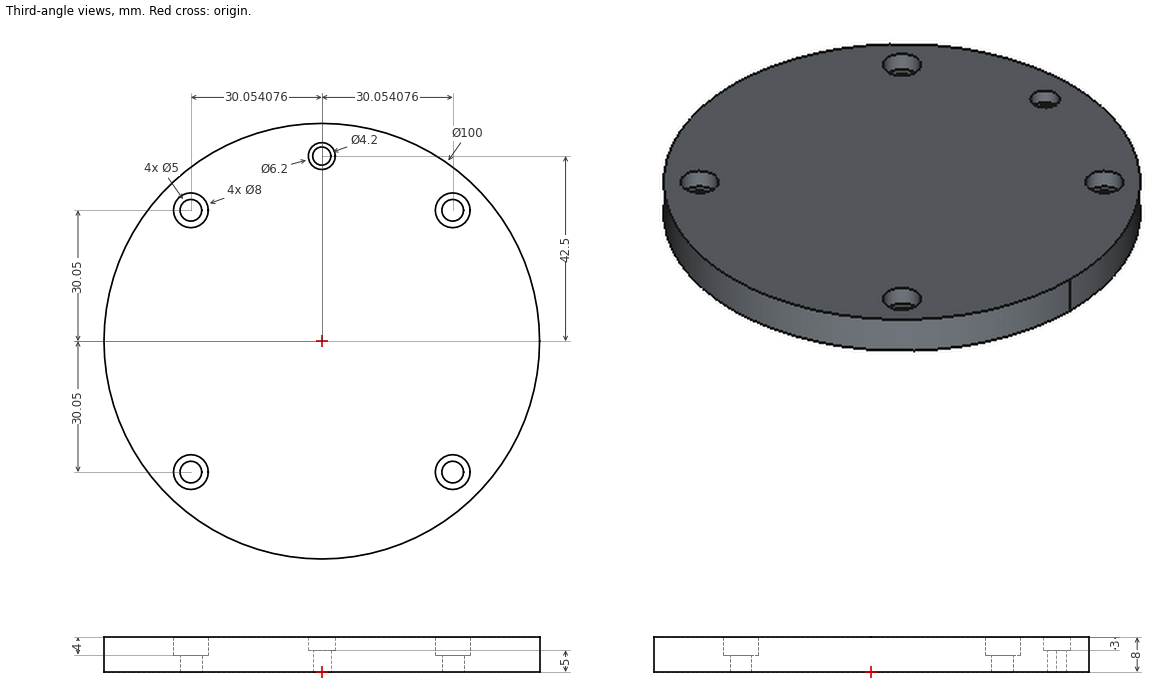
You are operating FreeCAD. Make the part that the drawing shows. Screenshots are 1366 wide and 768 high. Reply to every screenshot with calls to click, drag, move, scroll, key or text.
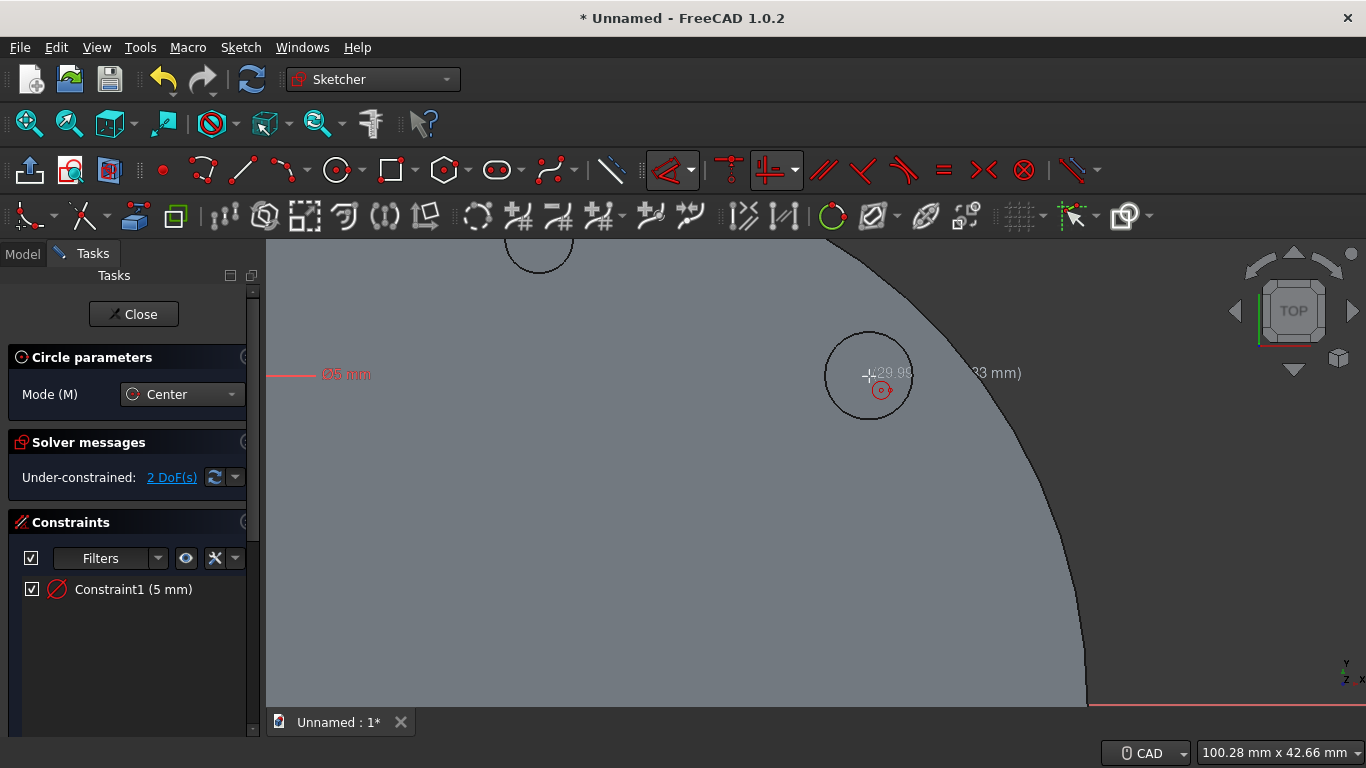
click(869, 376)
move(888, 356)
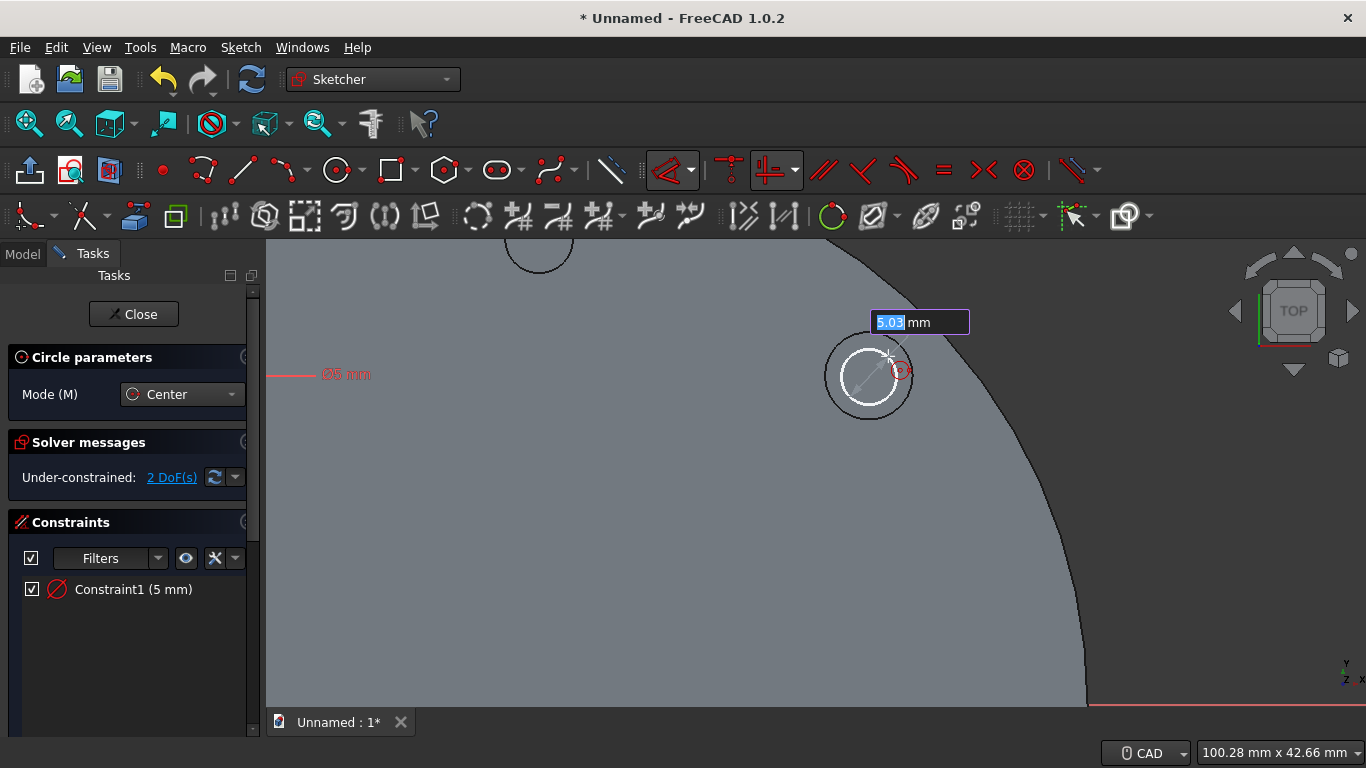
text(5)
key(Return)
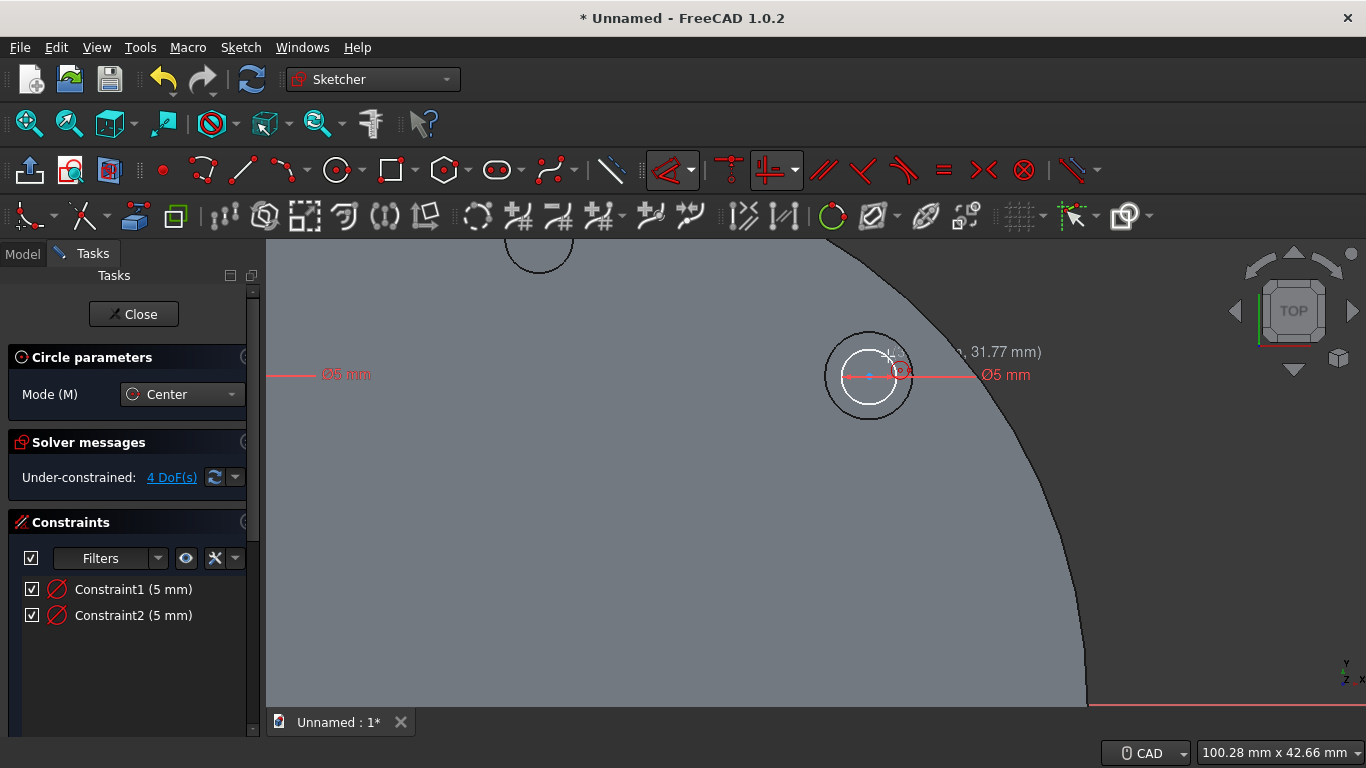
scroll(869, 376, down, 5)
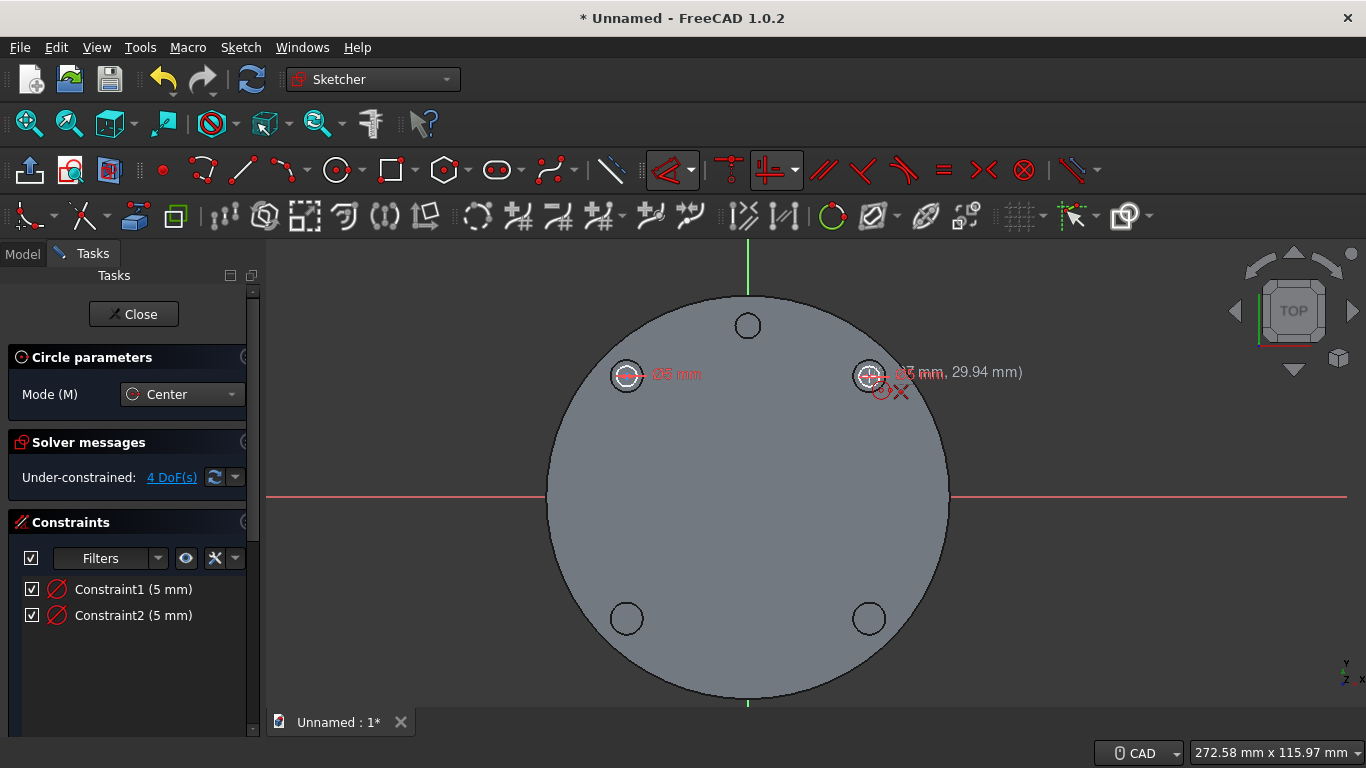
scroll(627, 619, up, 5)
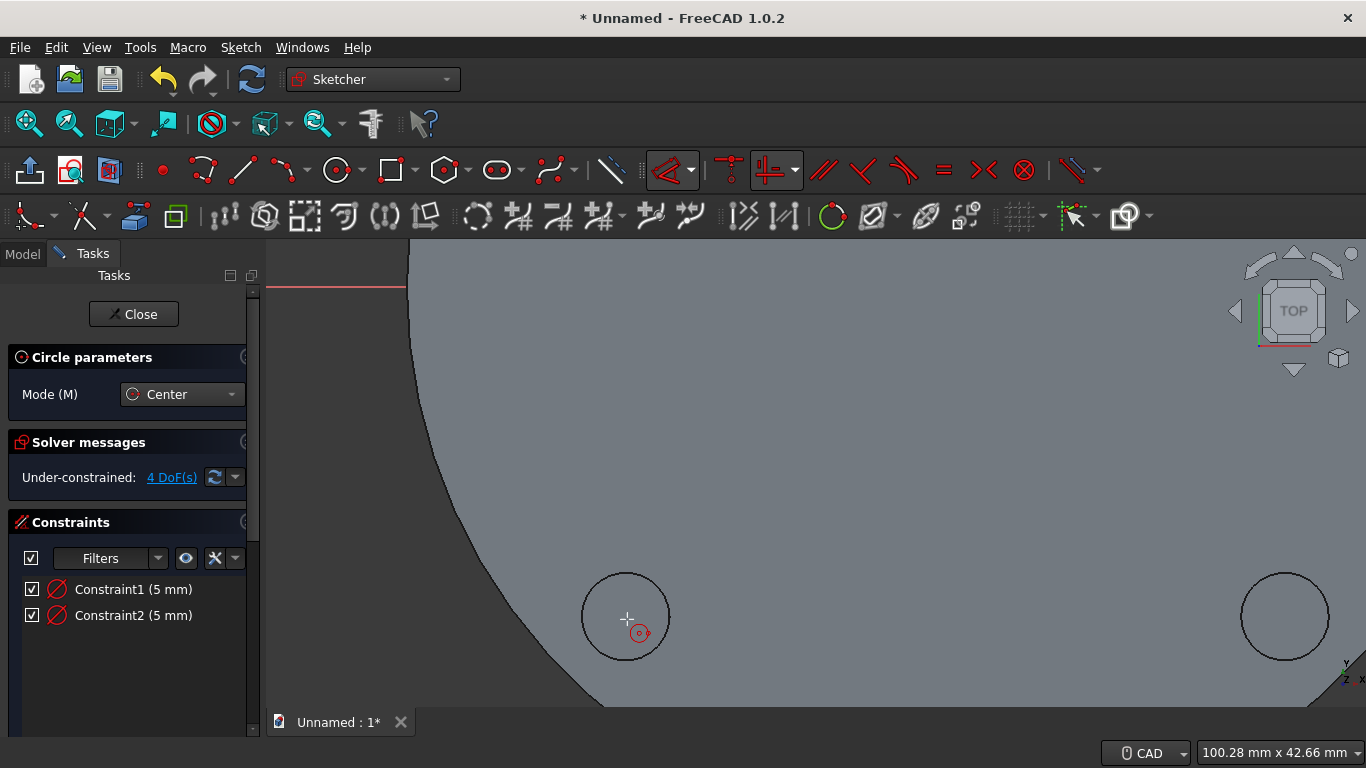
click(626, 617)
move(645, 597)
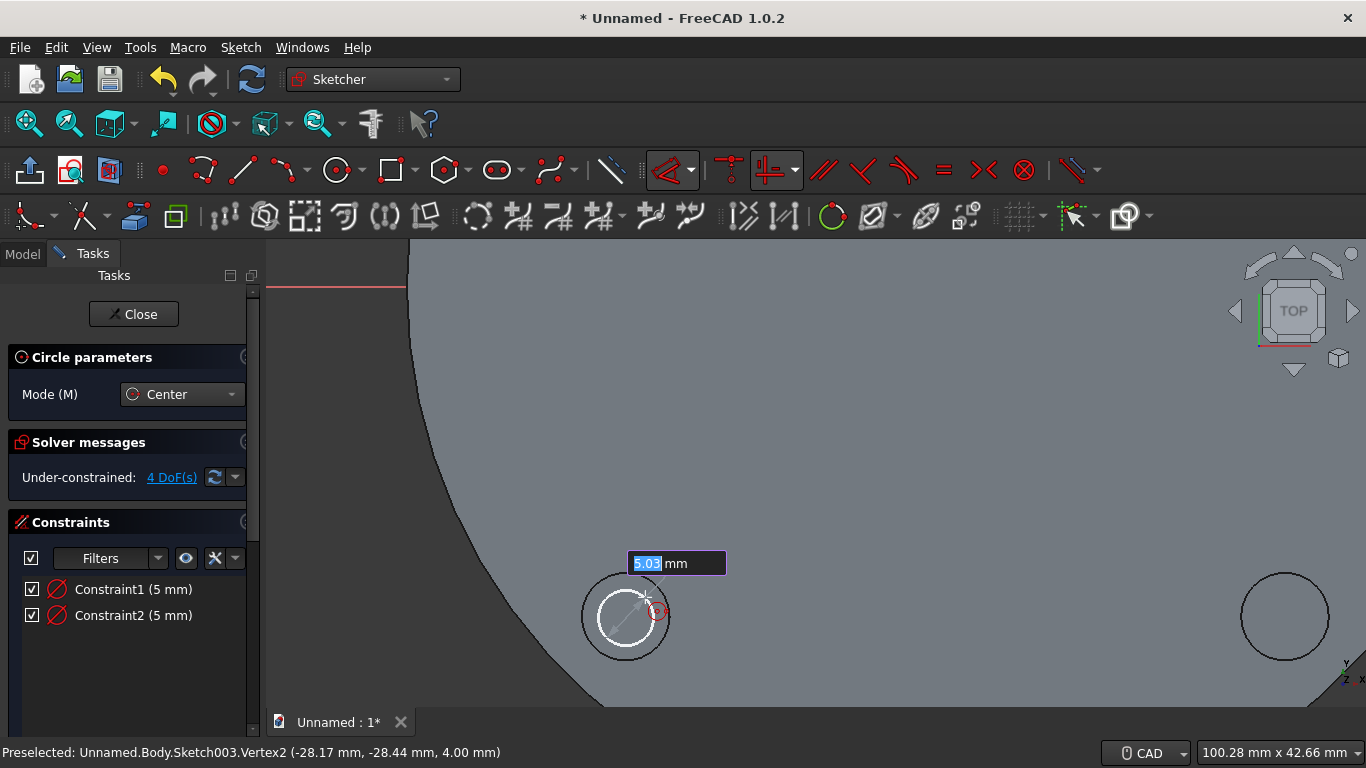
text(5)
key(Return)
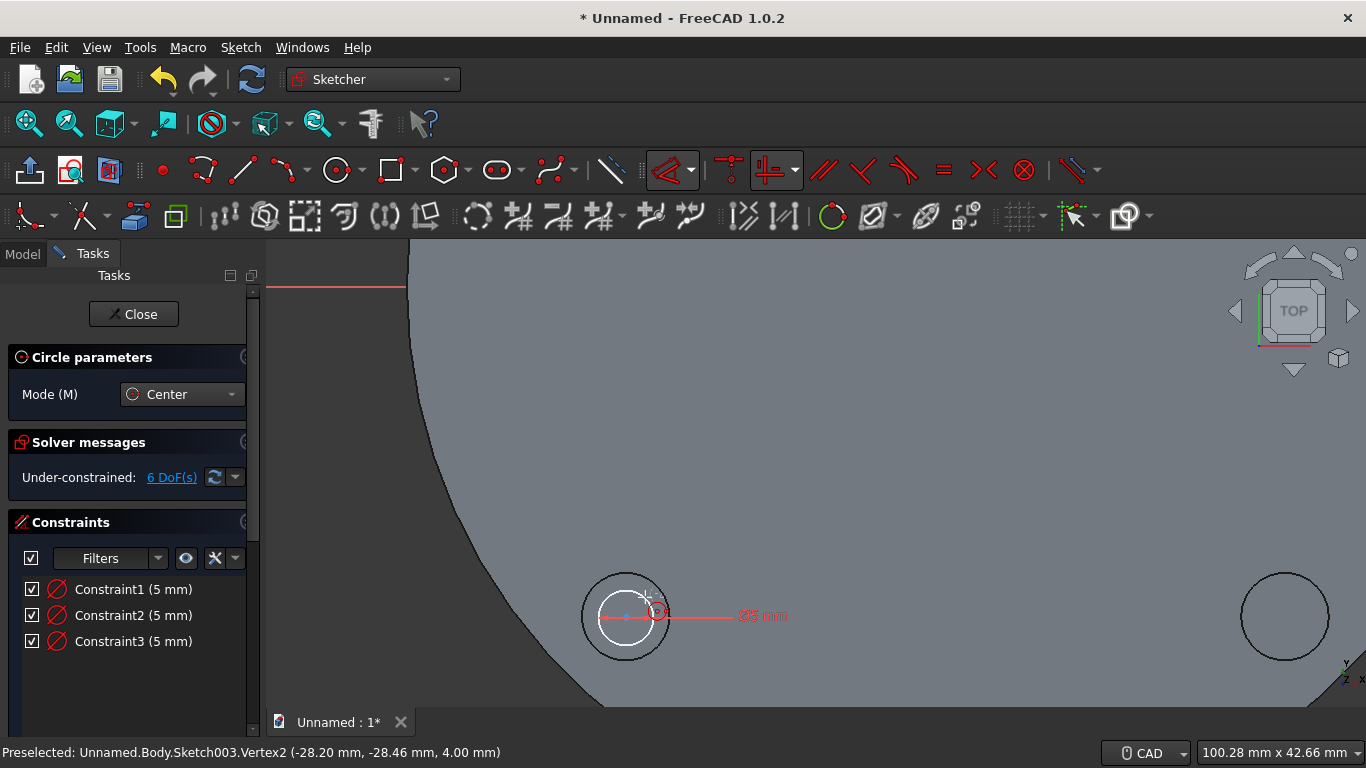
scroll(627, 620, down, 5)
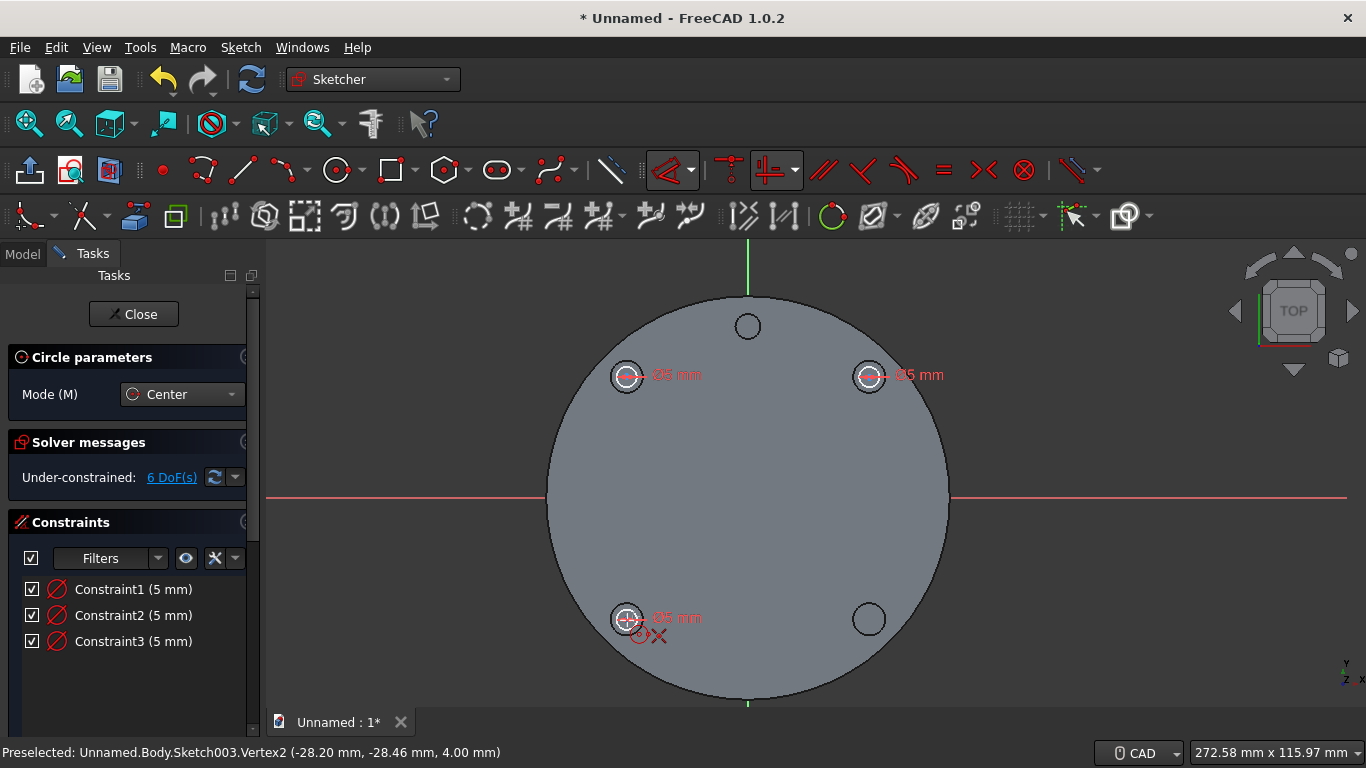
scroll(869, 619, up, 5)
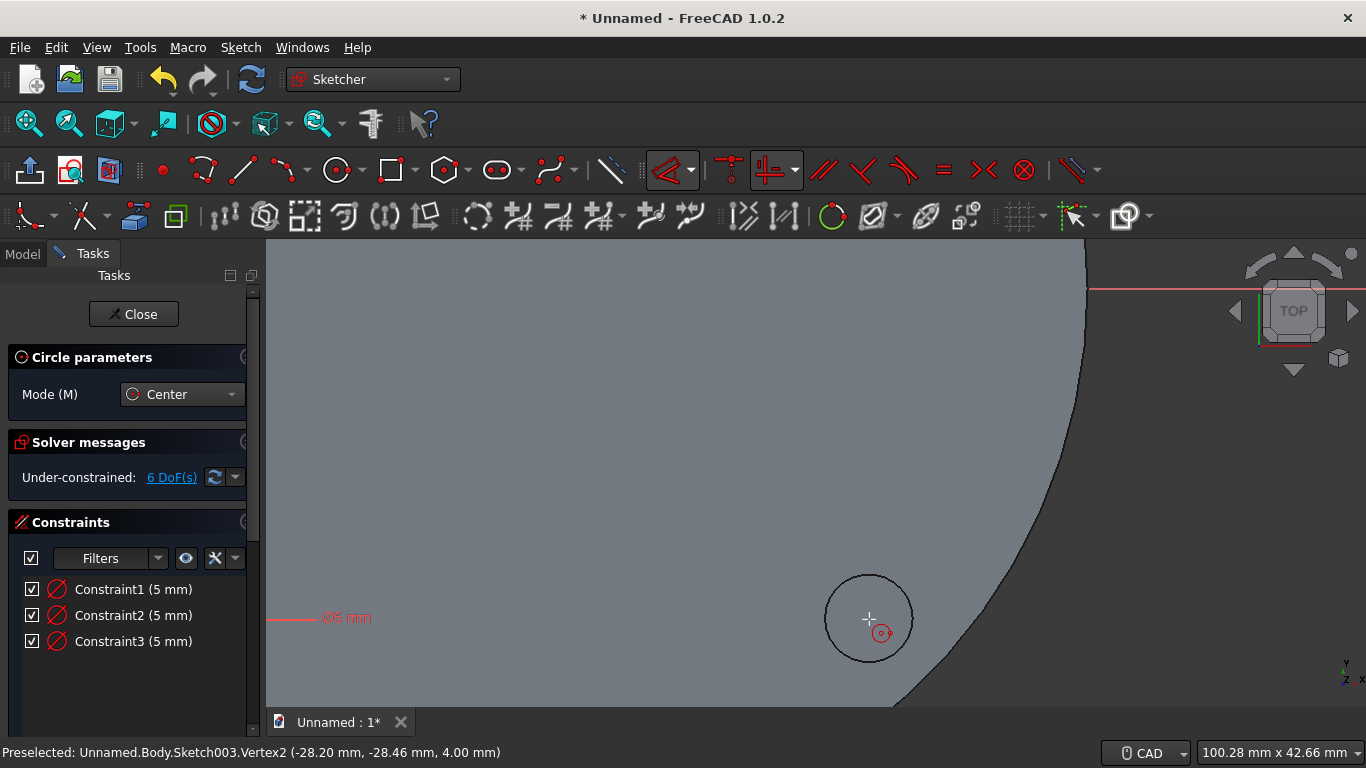
click(869, 618)
move(888, 599)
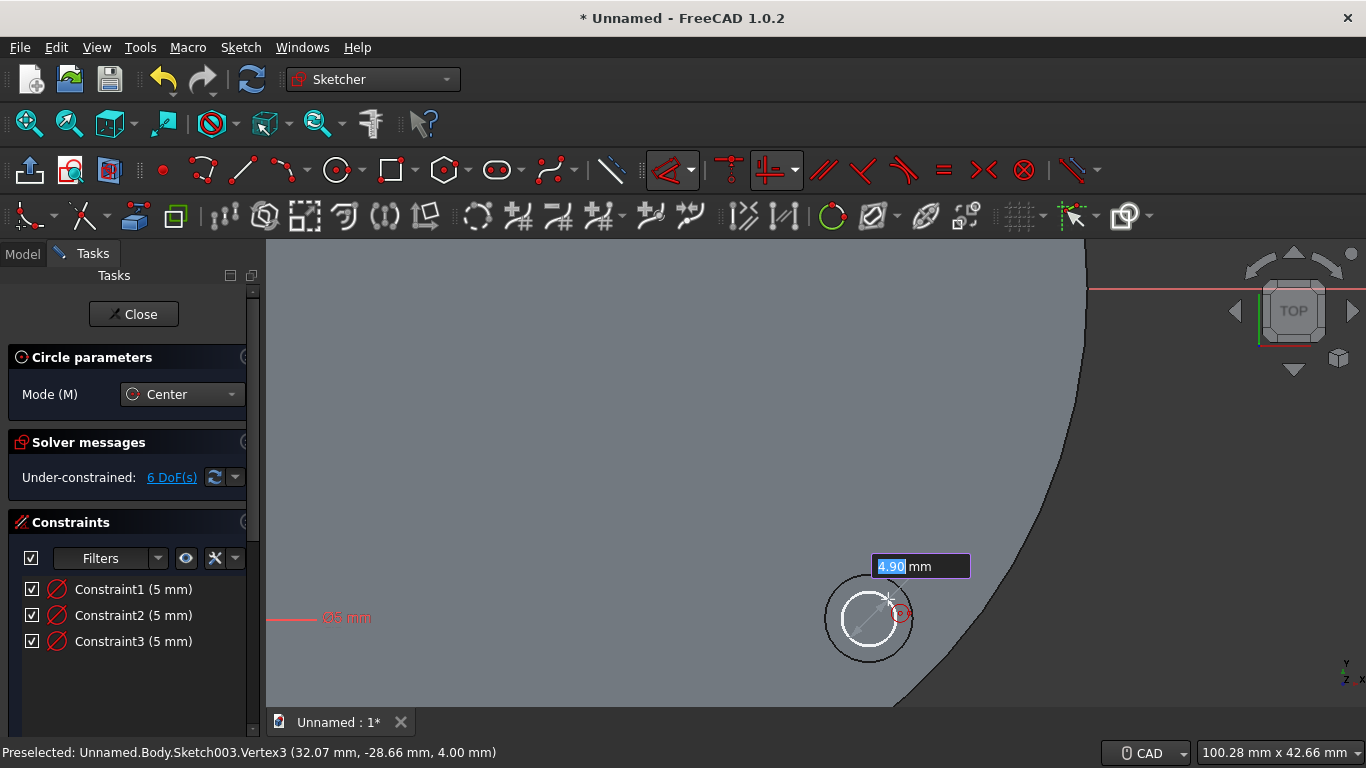
text(5)
key(Return)